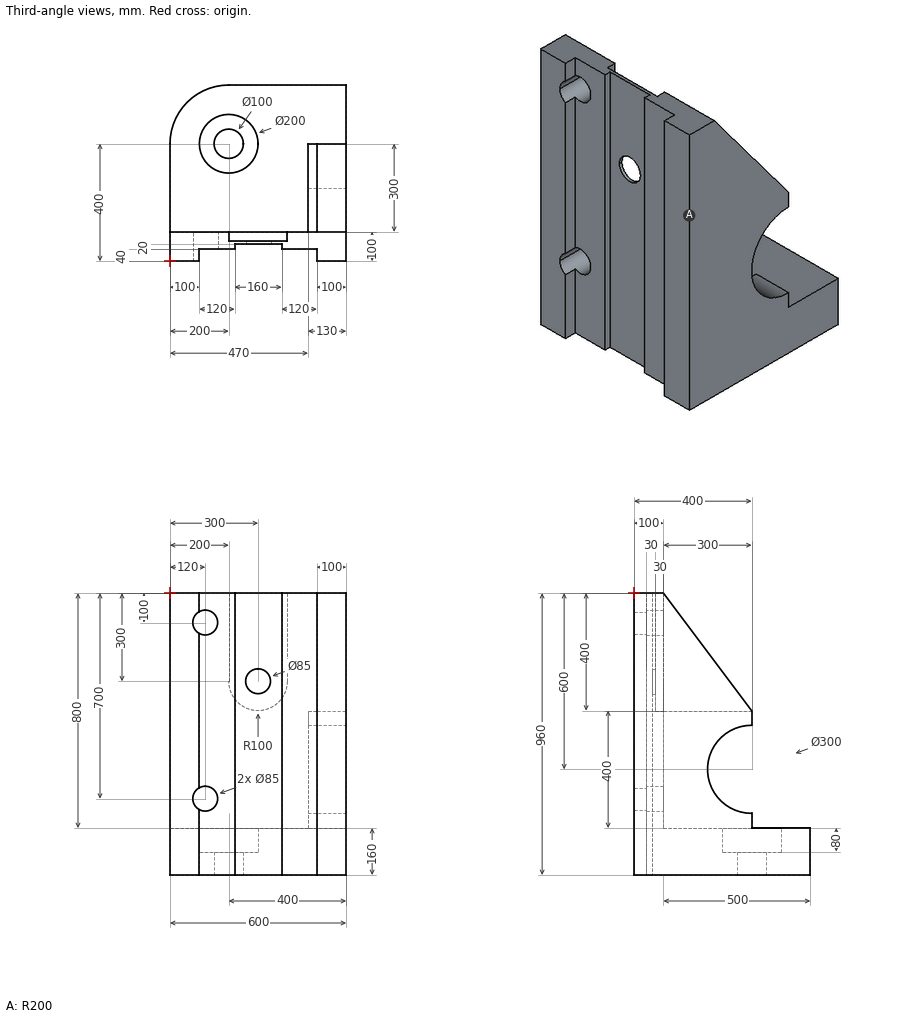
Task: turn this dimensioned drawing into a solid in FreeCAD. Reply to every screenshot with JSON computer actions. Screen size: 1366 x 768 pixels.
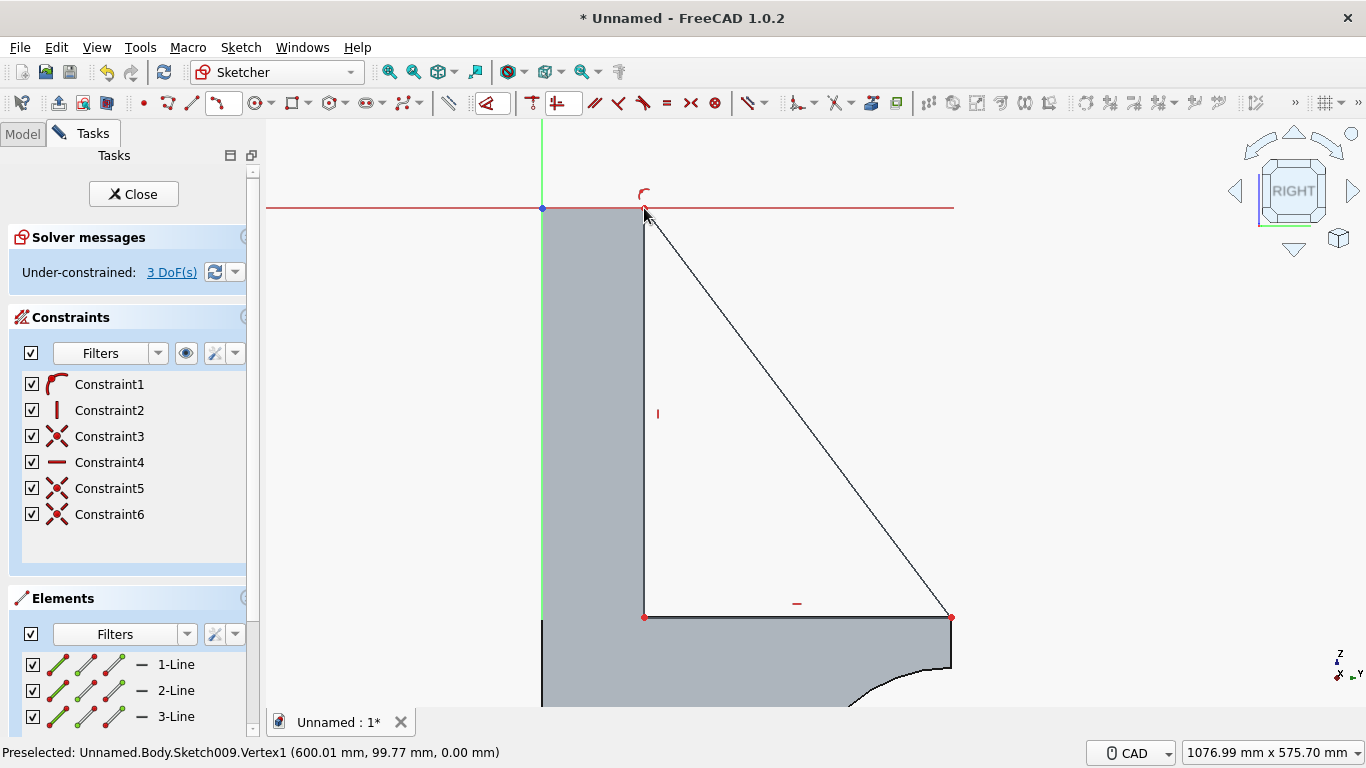
{"action": "left_click", "coordinate": [644, 331]}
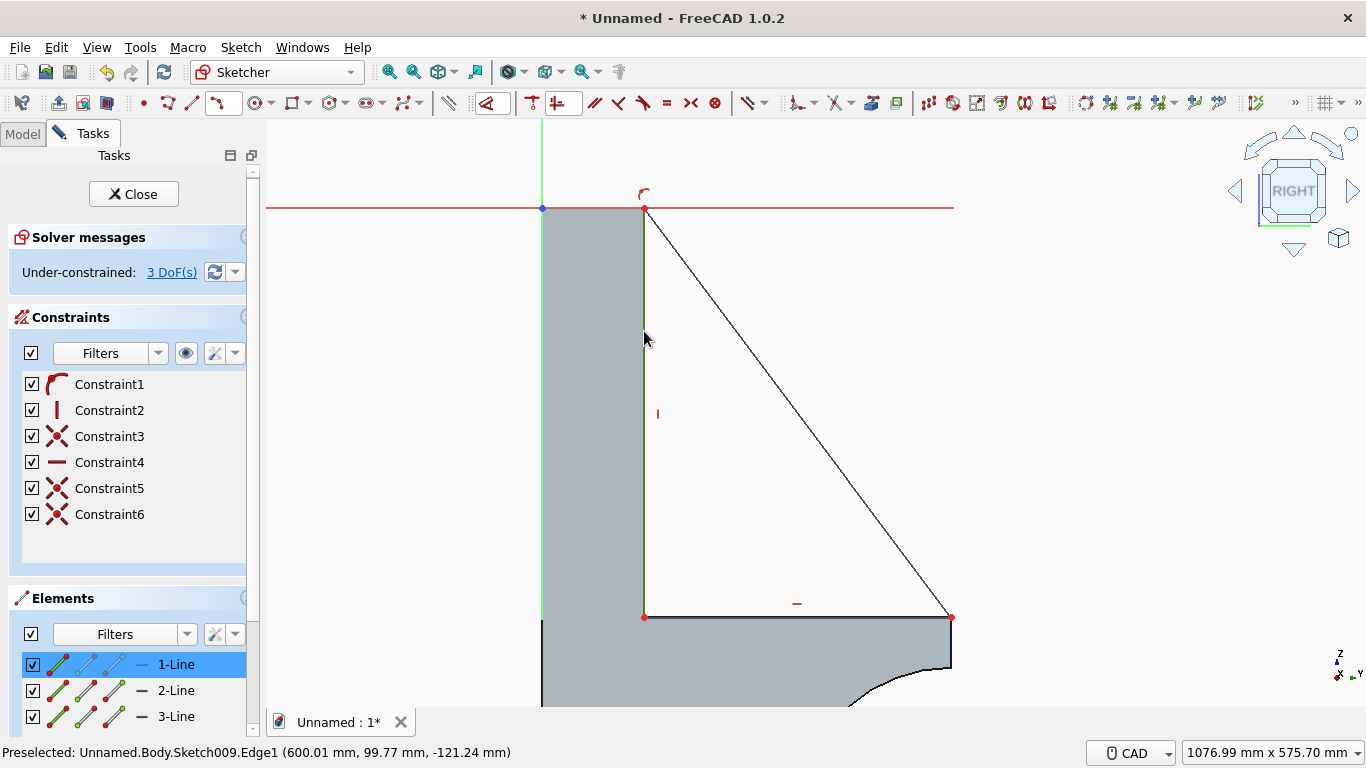
{"action": "key", "text": "i"}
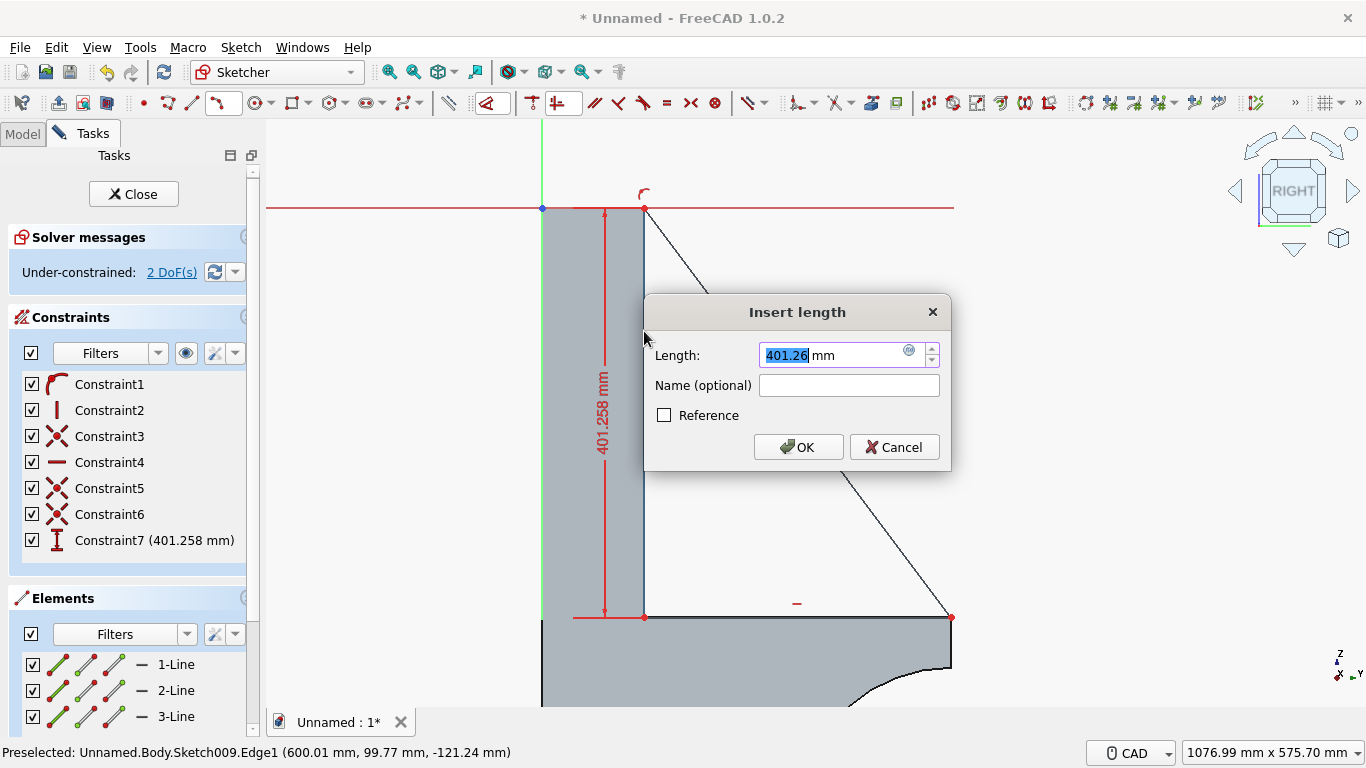
{"action": "type", "text": "400"}
{"action": "key", "text": "Return"}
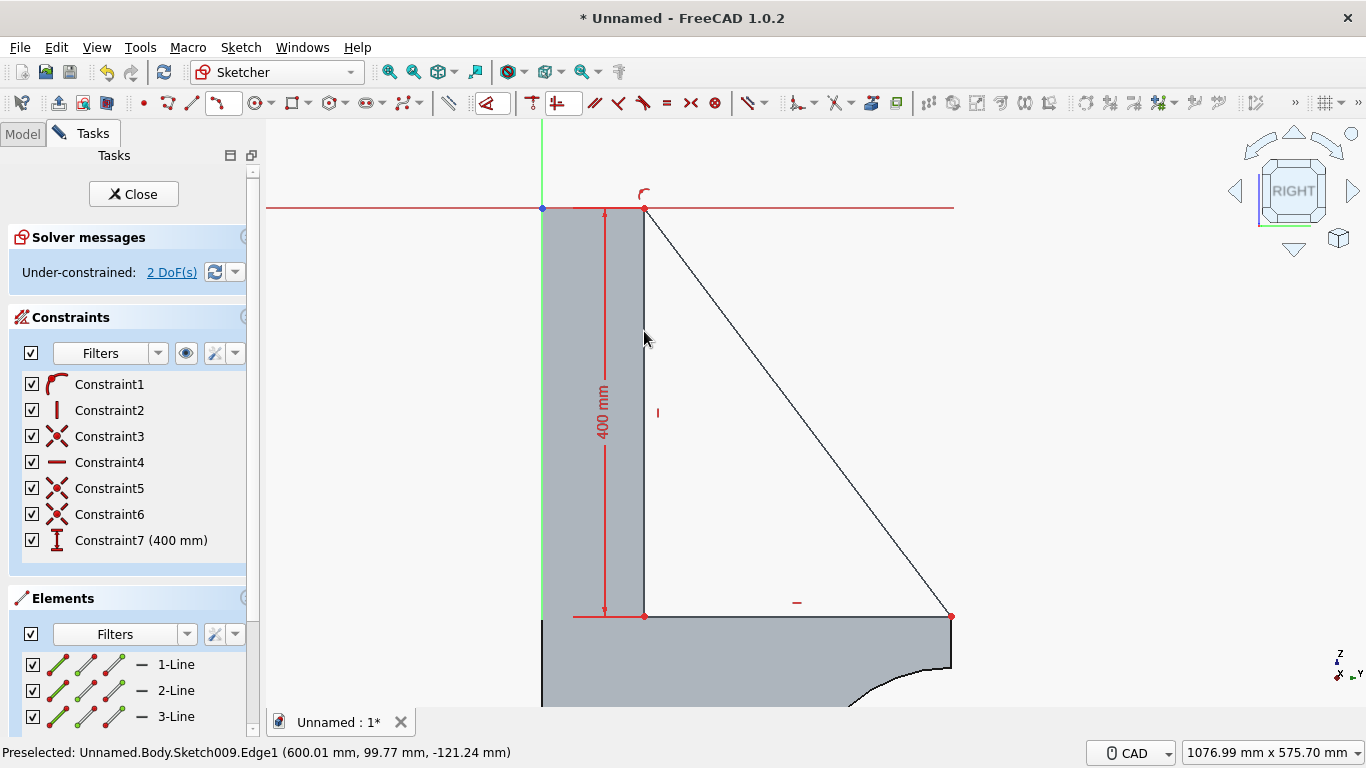
{"action": "left_click", "coordinate": [736, 617]}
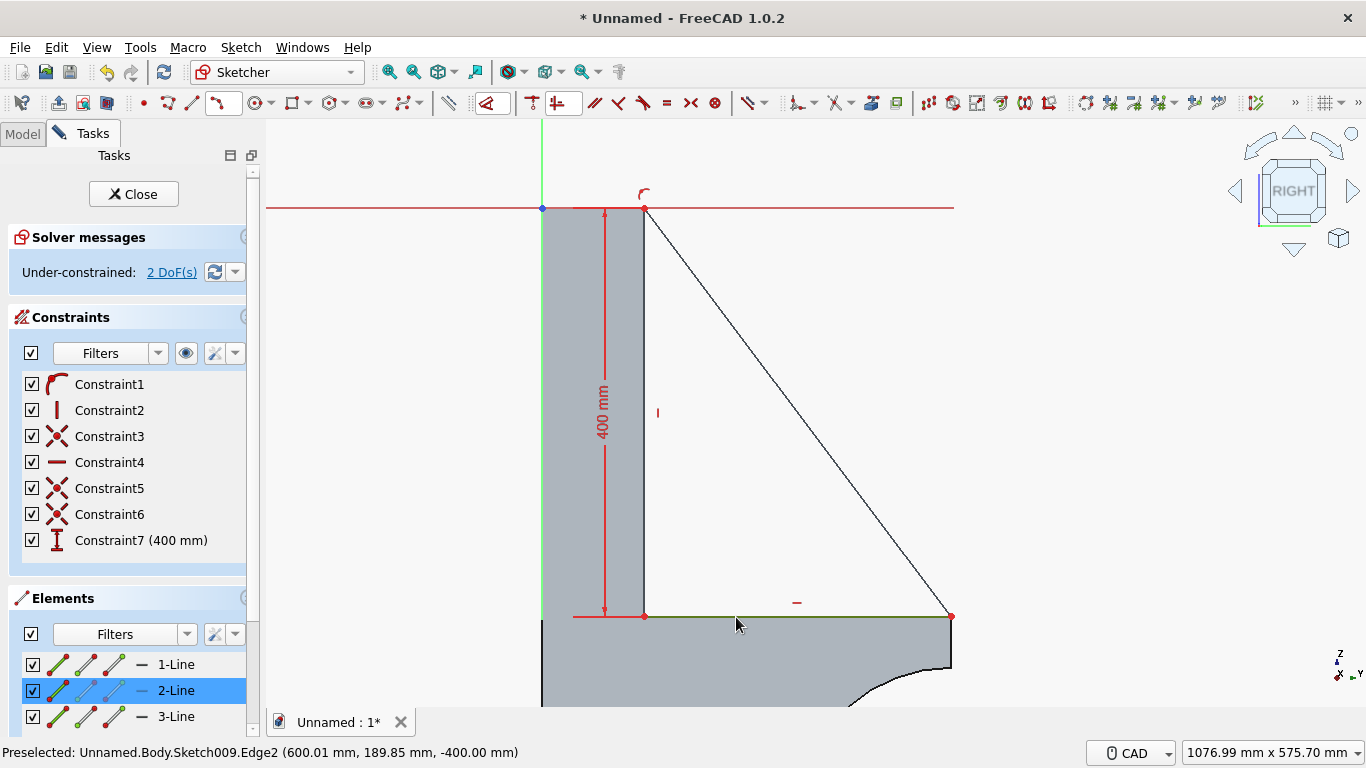
{"action": "left_click", "coordinate": [504, 104]}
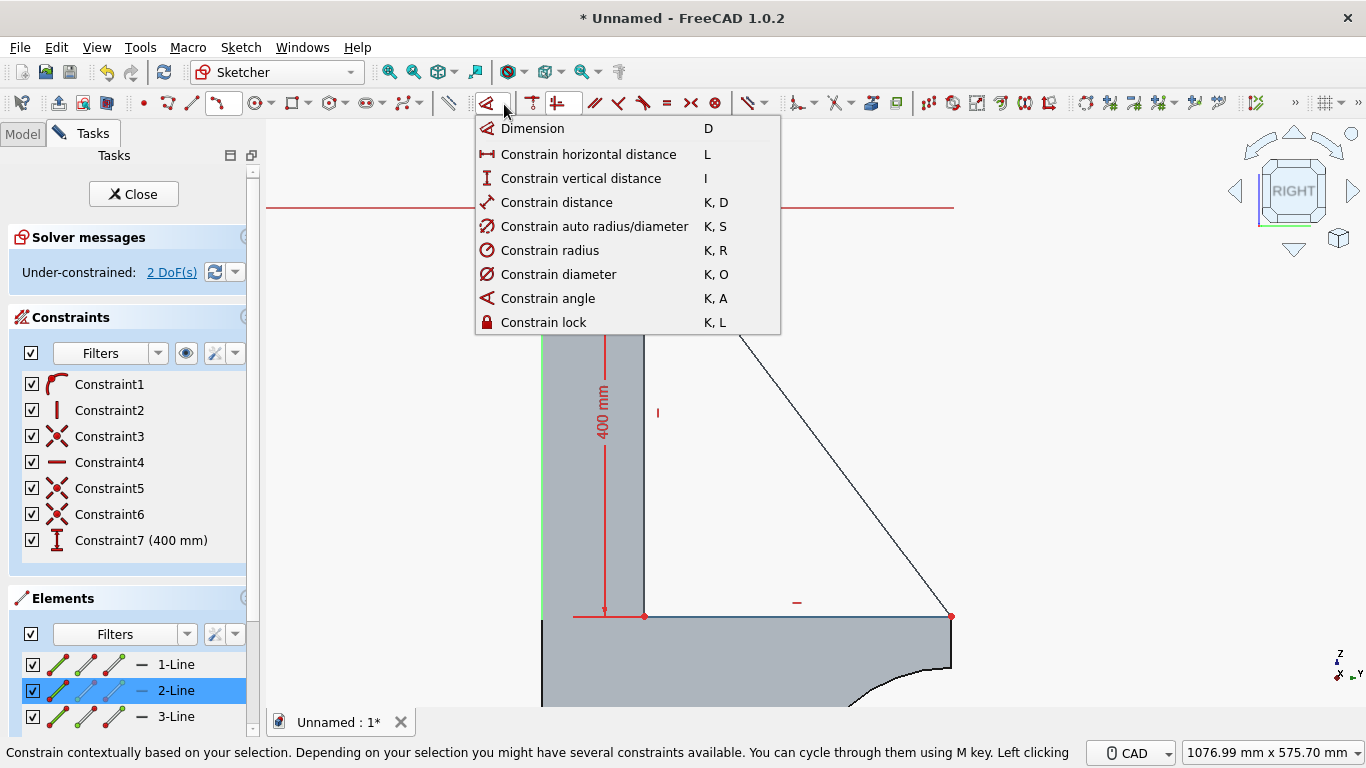
{"action": "left_click", "coordinate": [628, 154]}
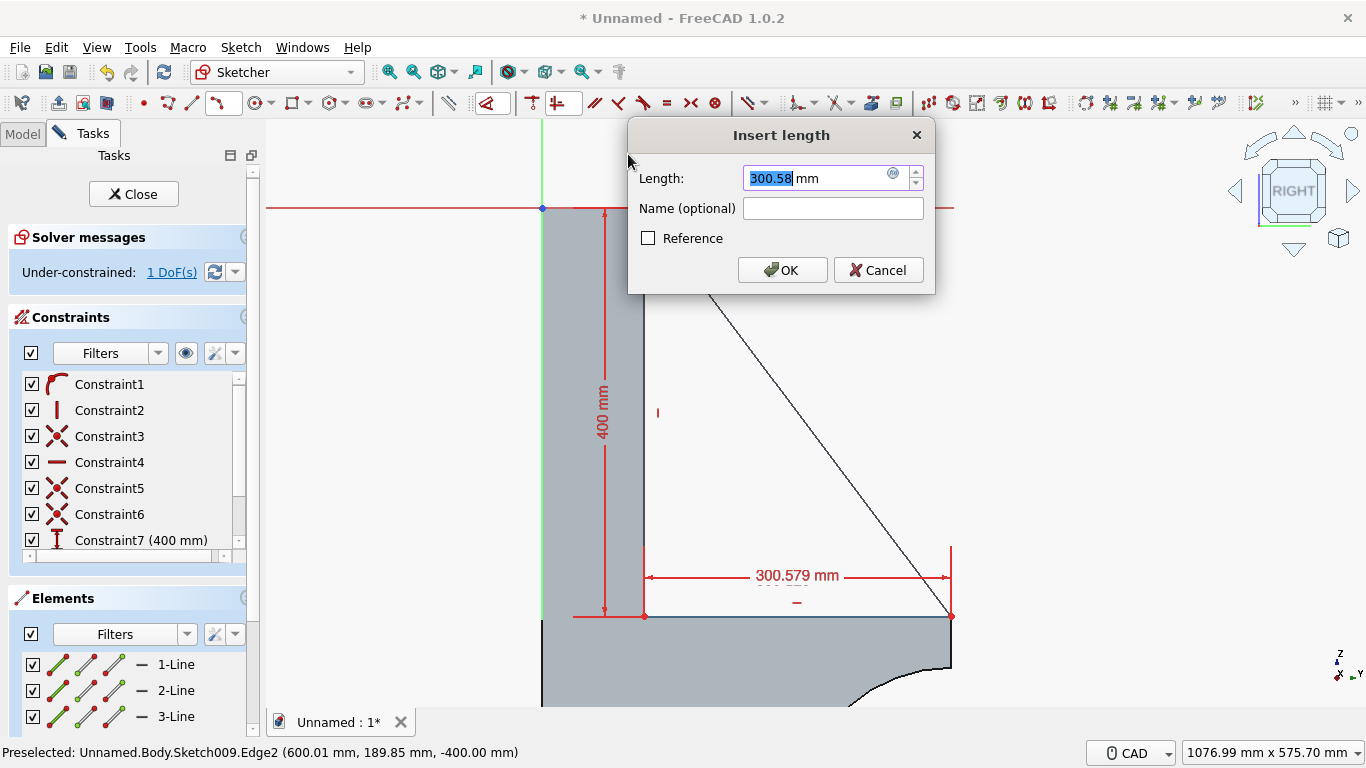
{"action": "type", "text": "300"}
{"action": "key", "text": "Return"}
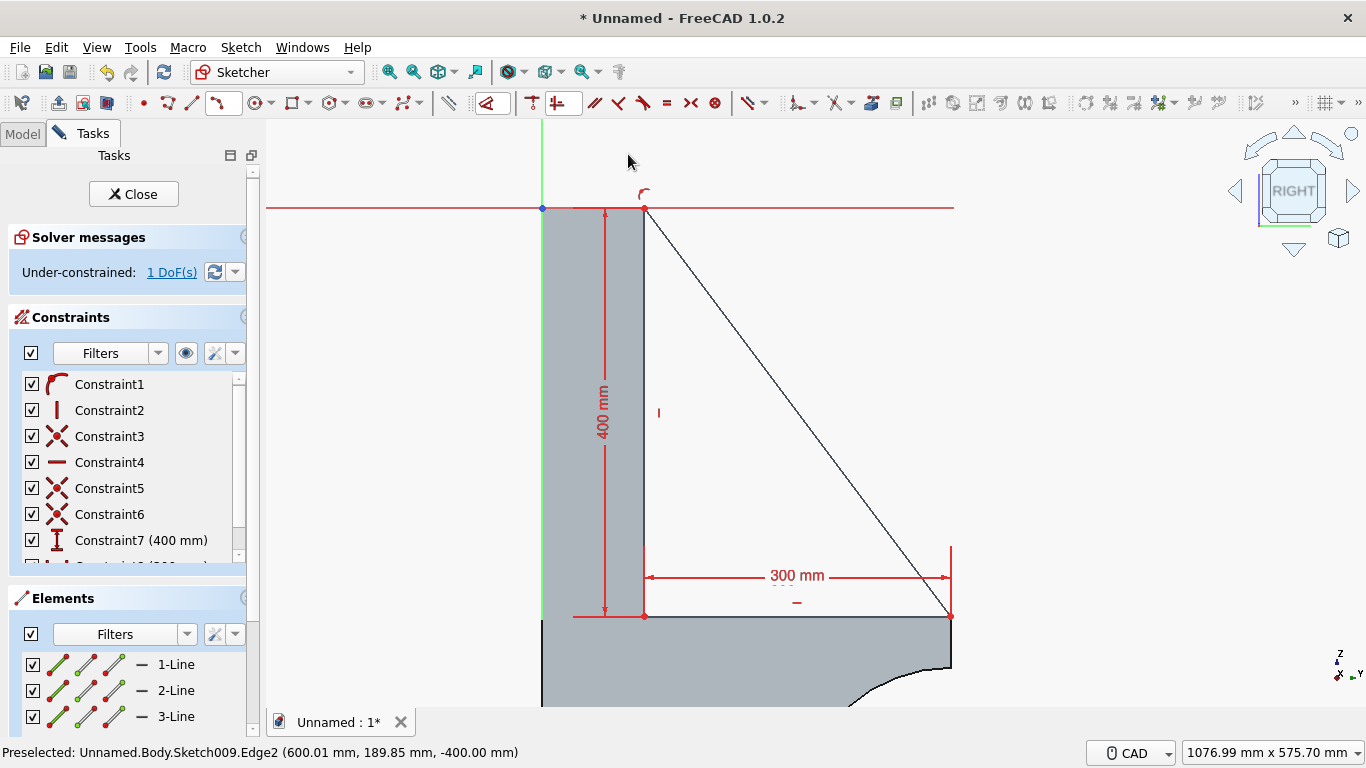
{"action": "left_click", "coordinate": [644, 208]}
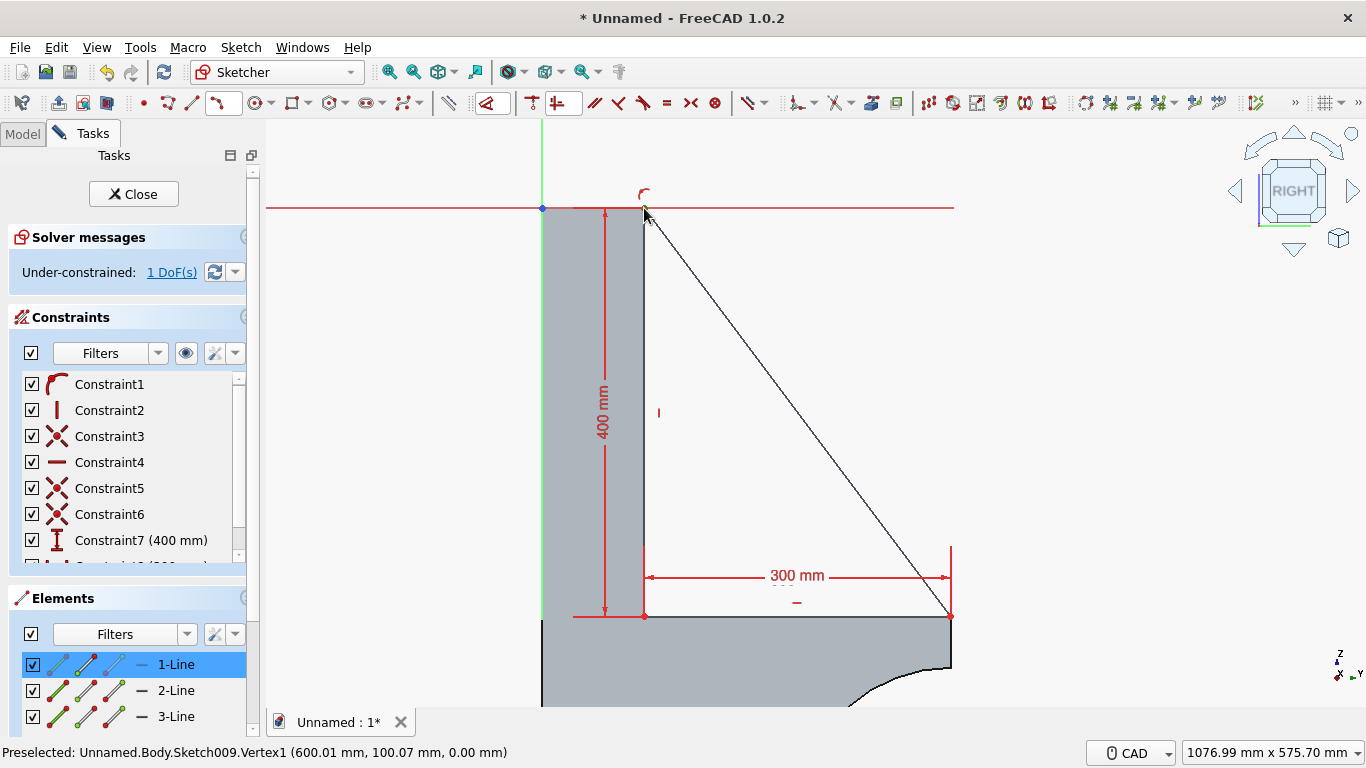
{"action": "left_click", "coordinate": [504, 104]}